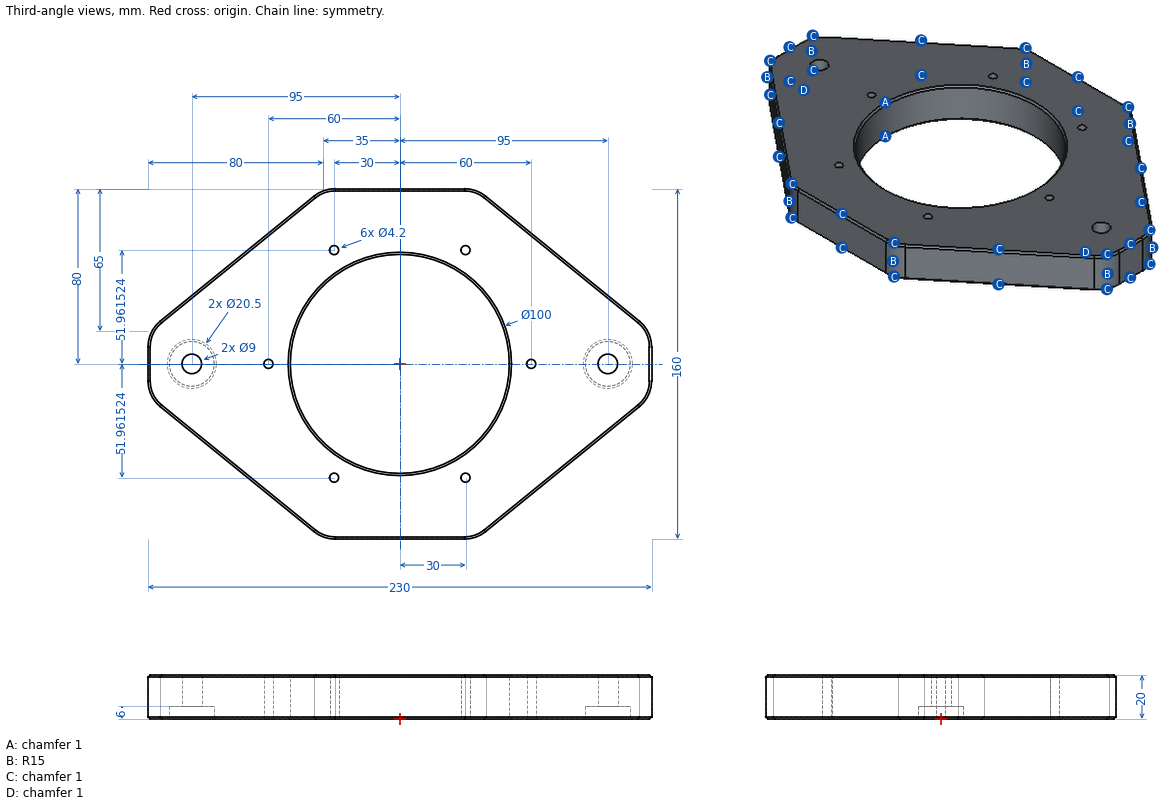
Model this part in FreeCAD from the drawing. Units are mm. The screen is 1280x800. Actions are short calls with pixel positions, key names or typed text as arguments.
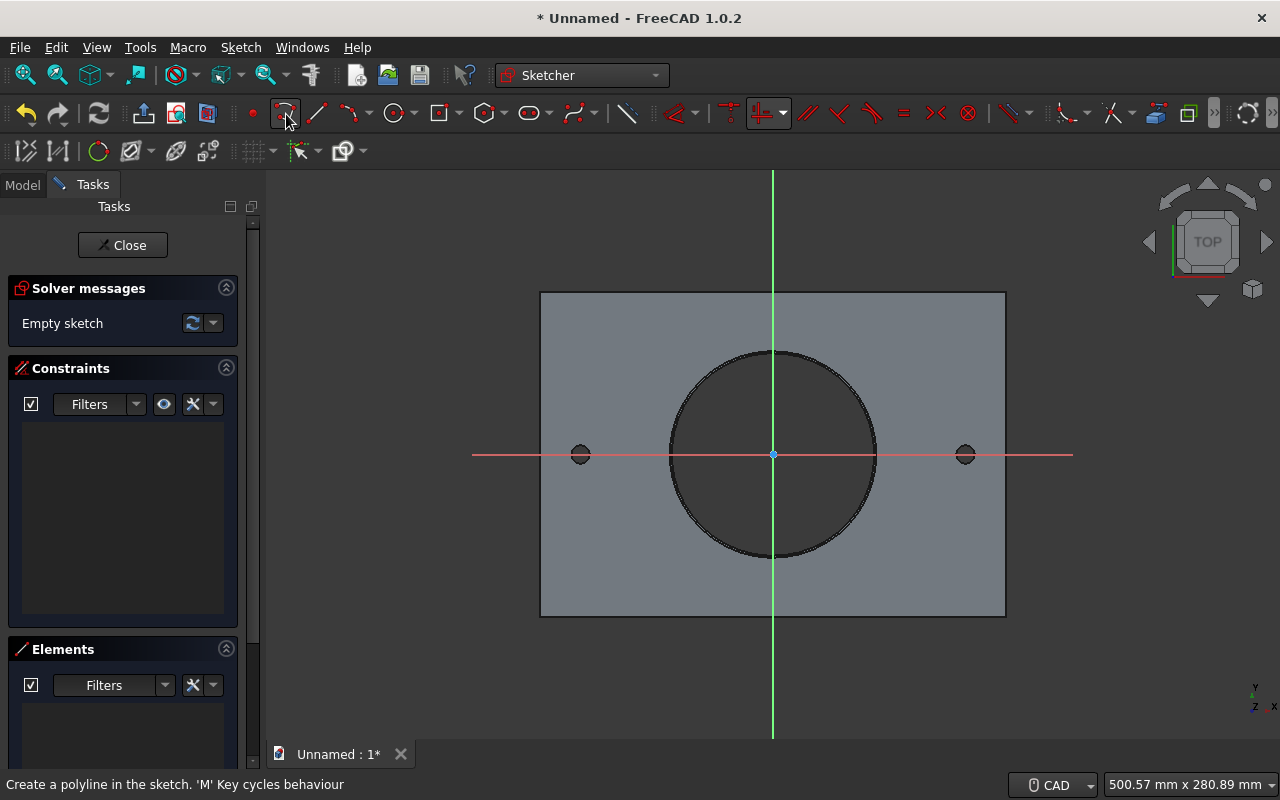
click(702, 292)
click(540, 292)
click(540, 424)
click(702, 293)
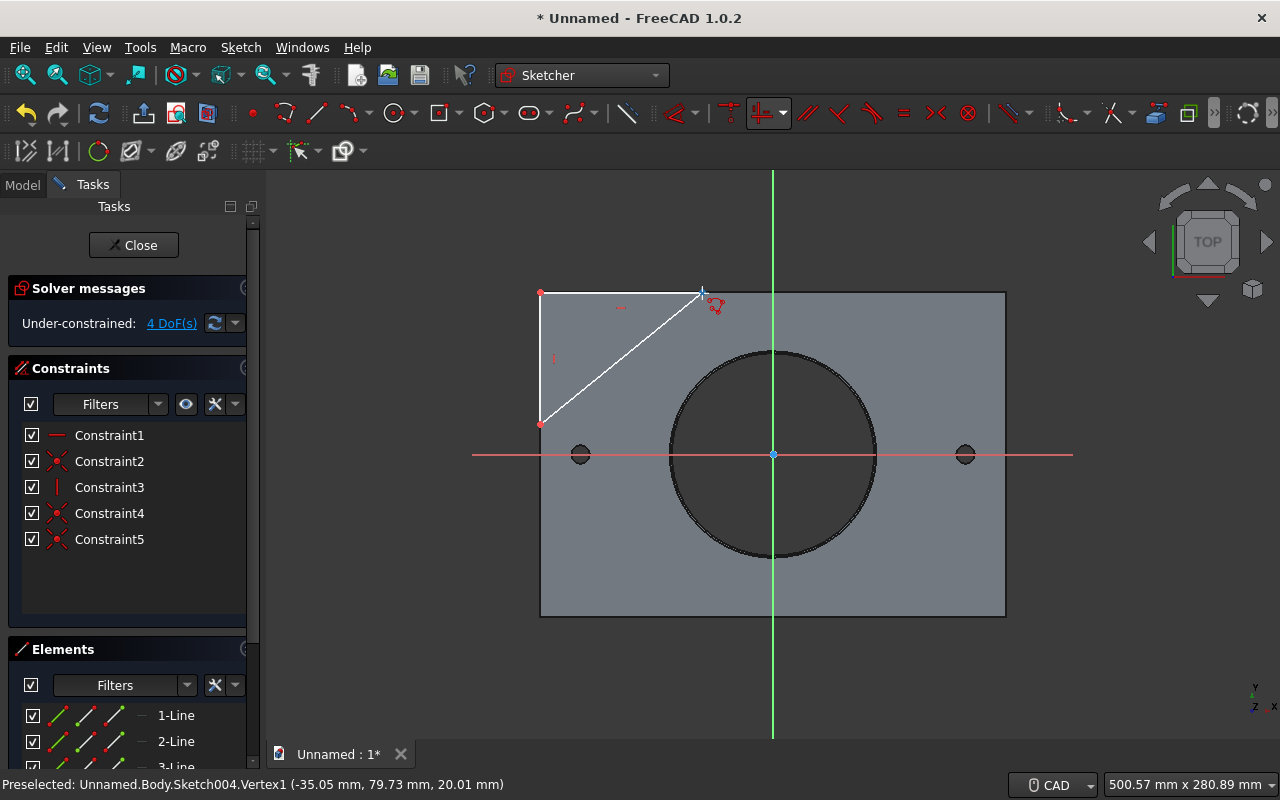
click(844, 292)
click(1006, 424)
click(1006, 292)
click(844, 293)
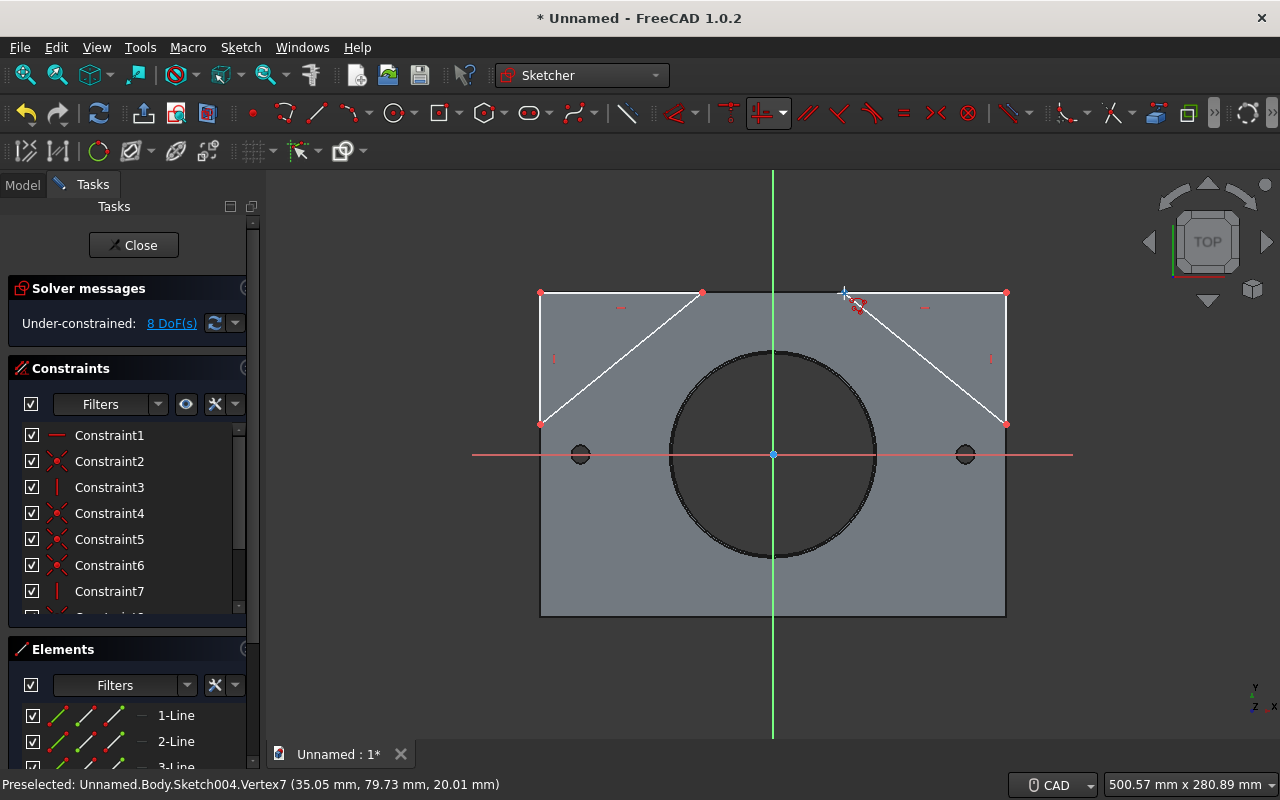
click(702, 617)
click(540, 485)
click(540, 617)
click(702, 618)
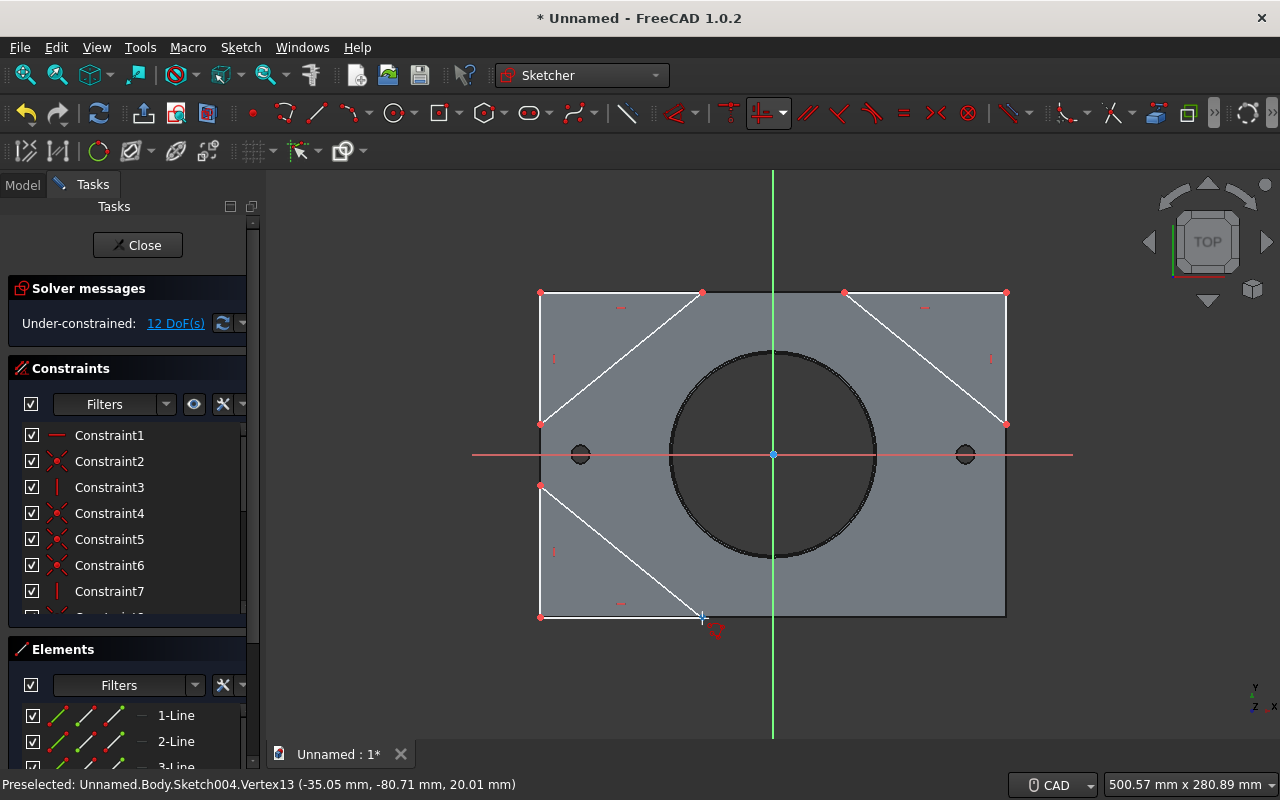
click(844, 617)
click(1006, 617)
click(1006, 485)
click(844, 618)
key(Escape)
key(Escape)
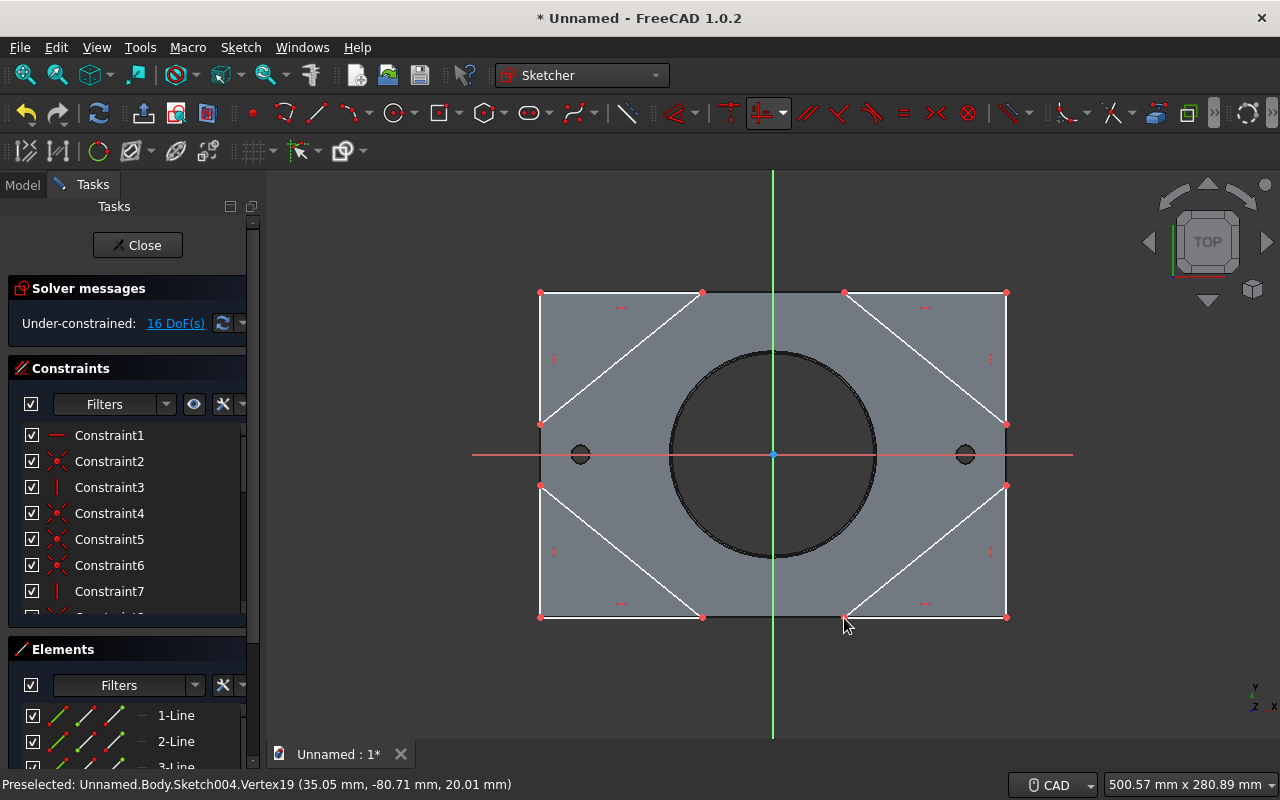
click(702, 293)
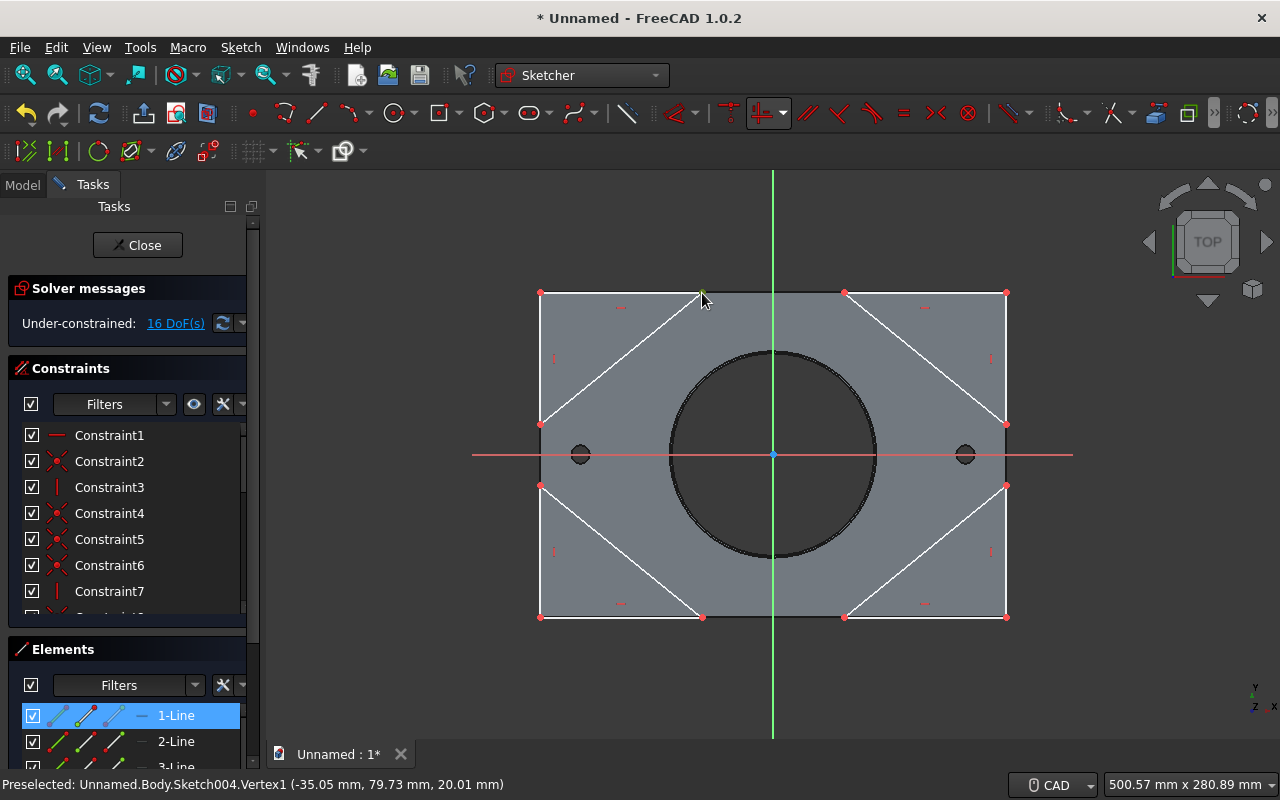
click(844, 293)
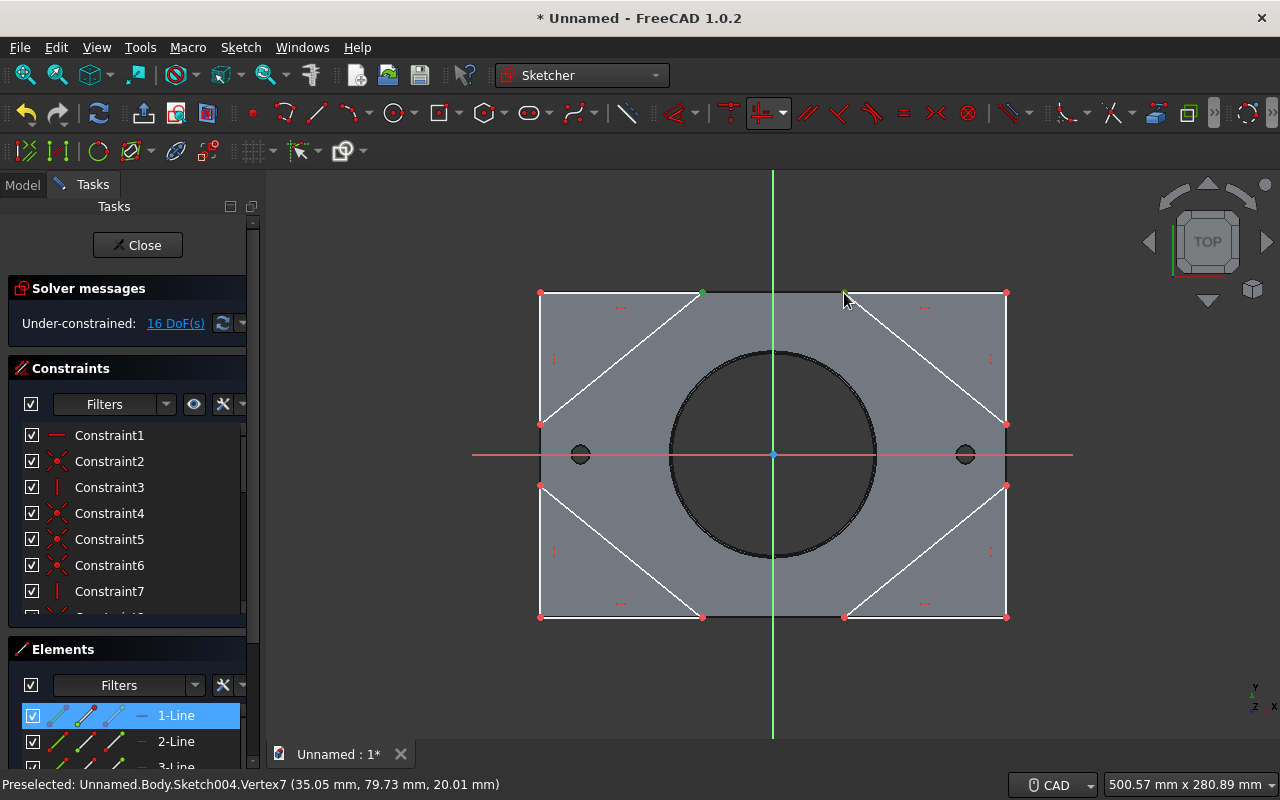
click(773, 674)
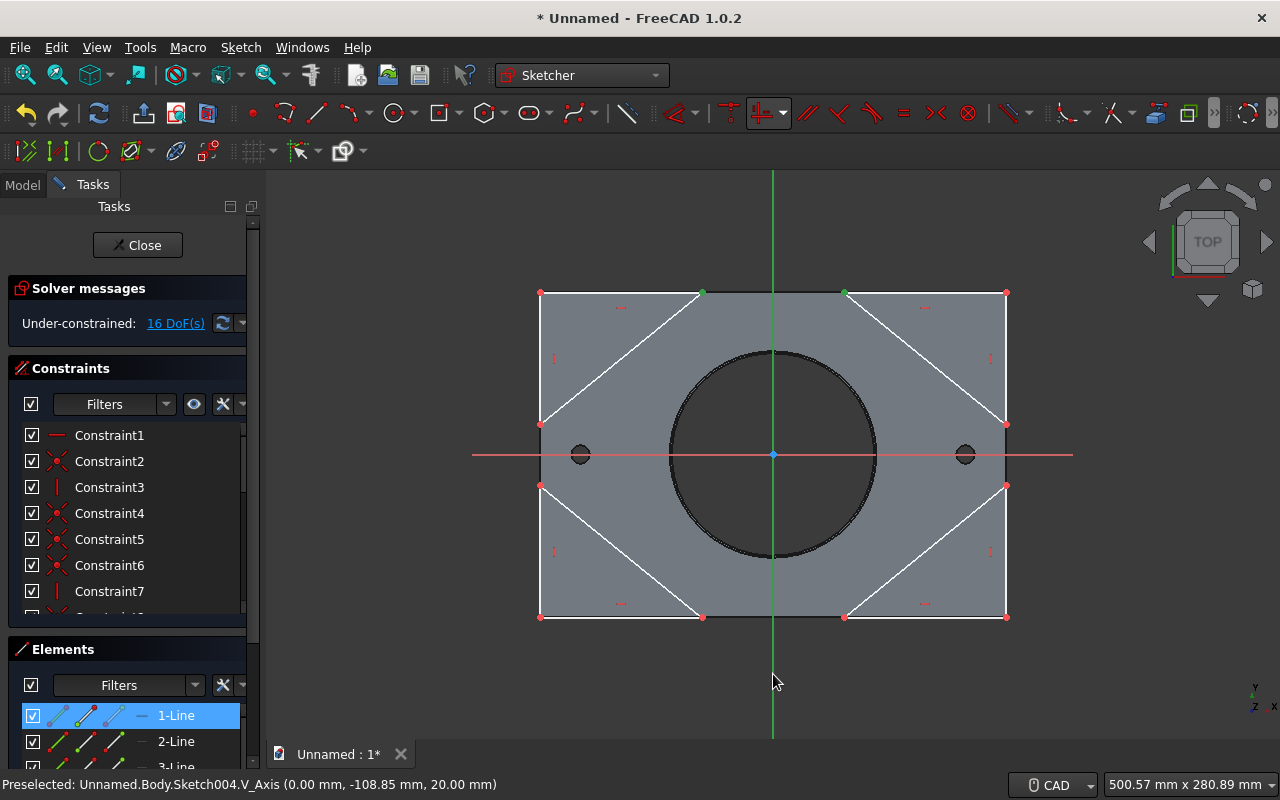
click(936, 114)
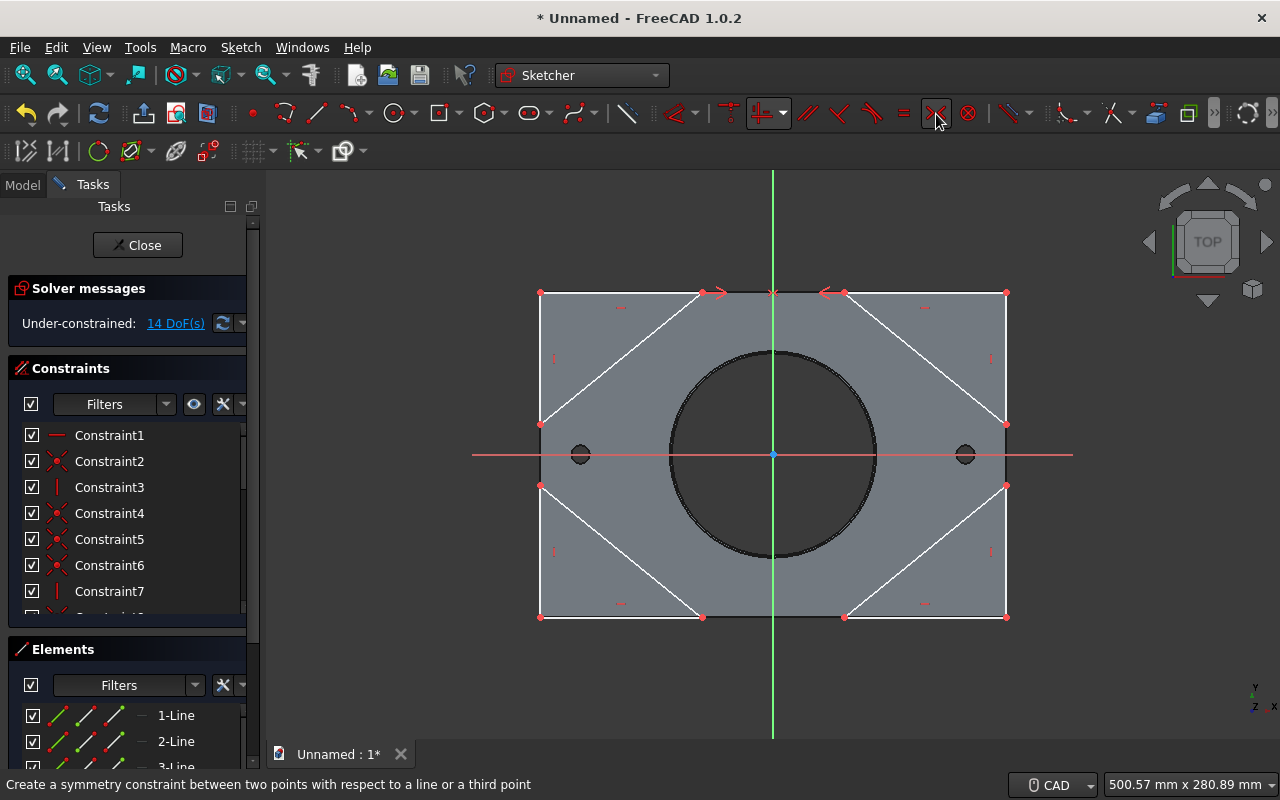
click(540, 425)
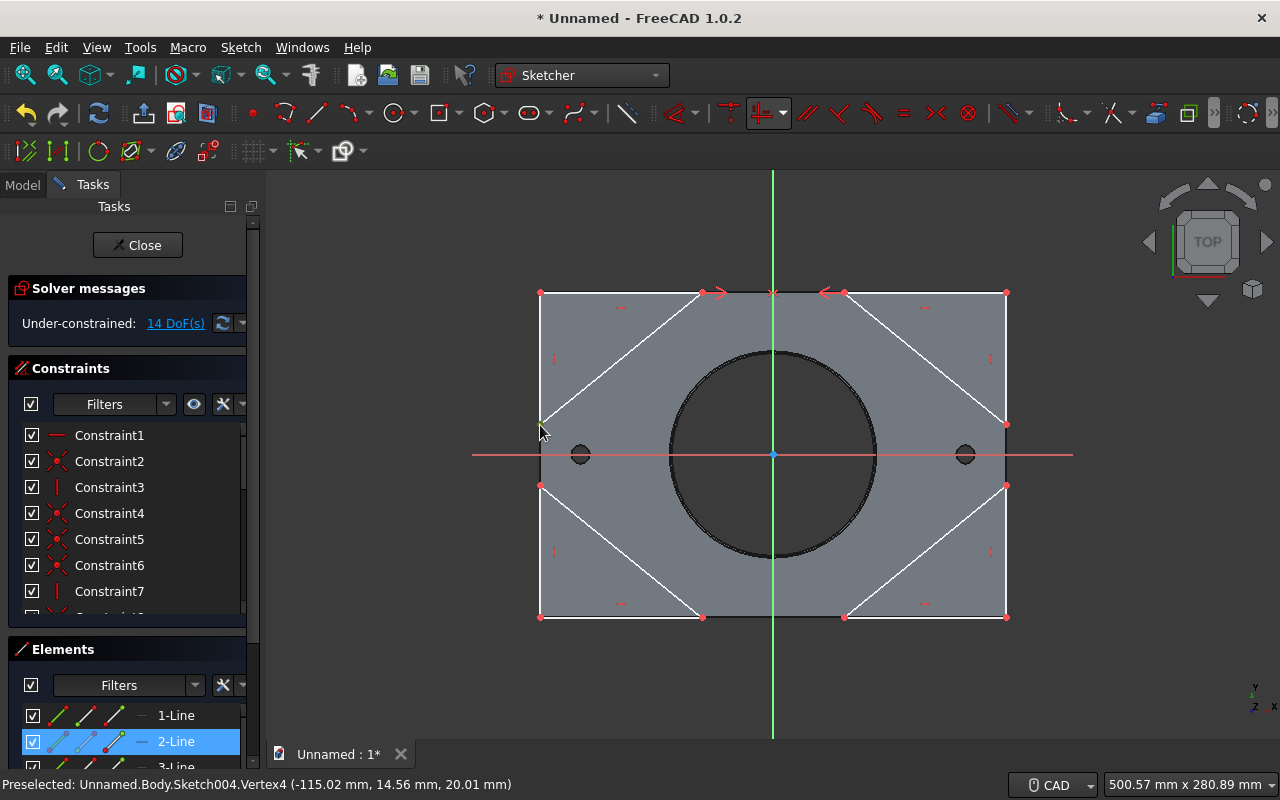
click(1006, 425)